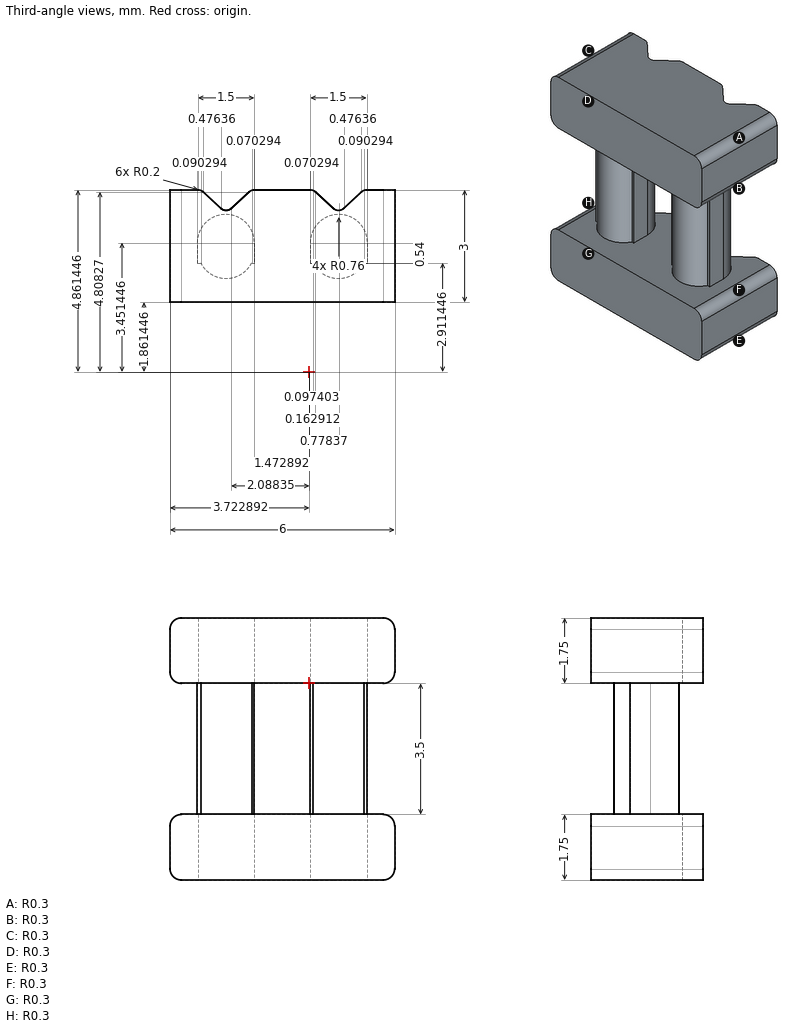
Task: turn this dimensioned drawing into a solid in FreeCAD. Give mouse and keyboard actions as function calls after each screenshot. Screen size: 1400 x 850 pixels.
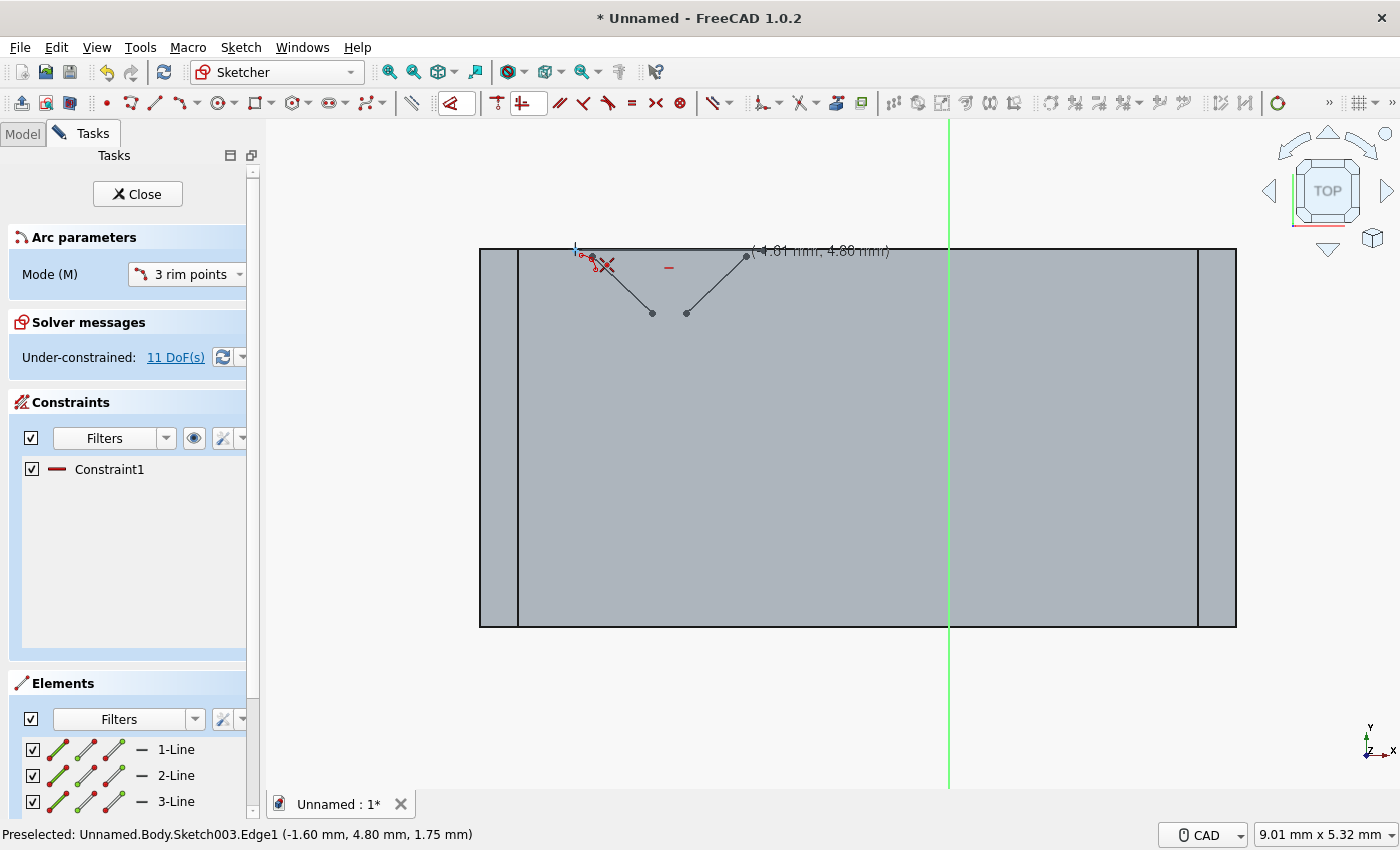
click(576, 250)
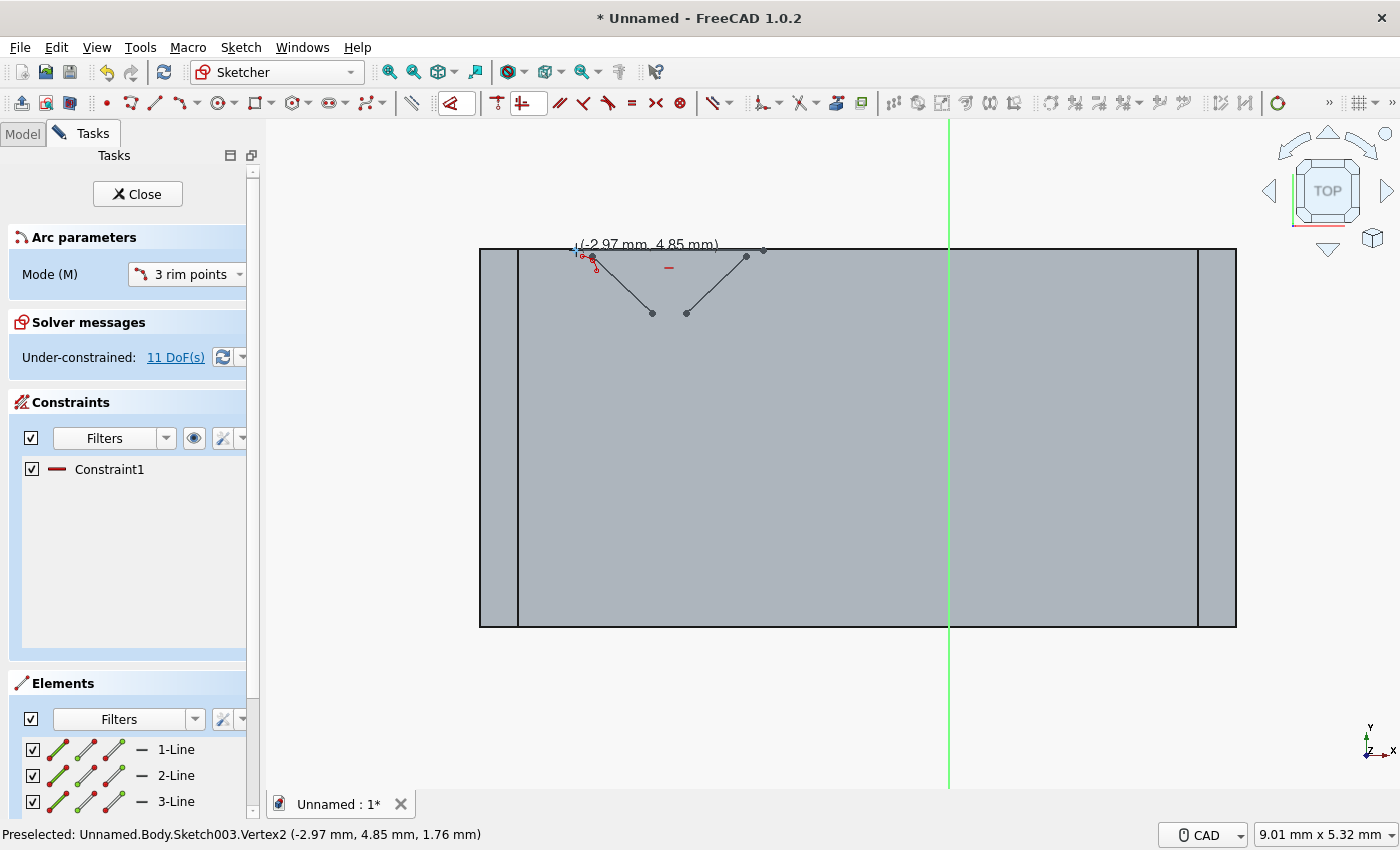
scroll(592, 256, up, 5)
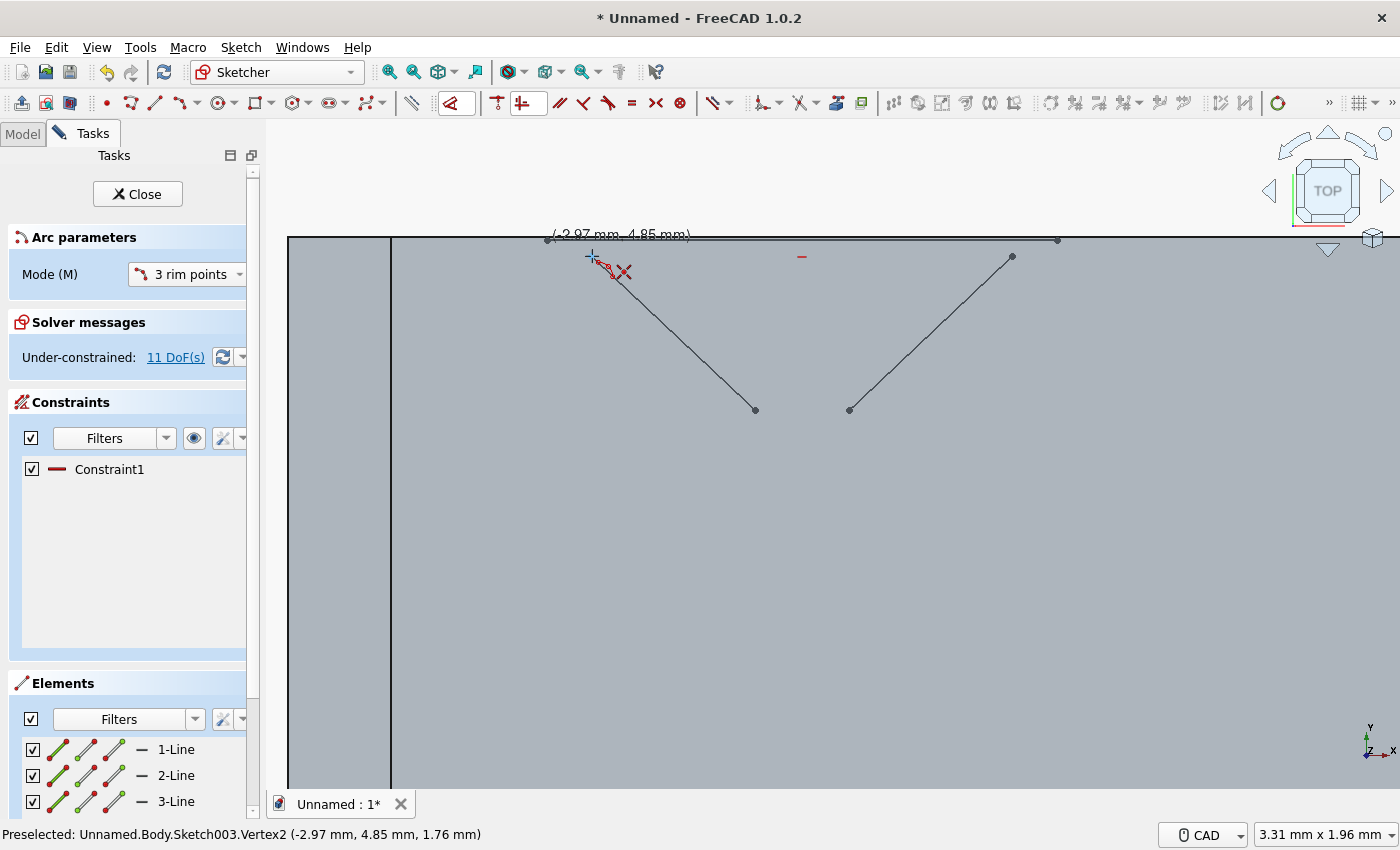
click(592, 256)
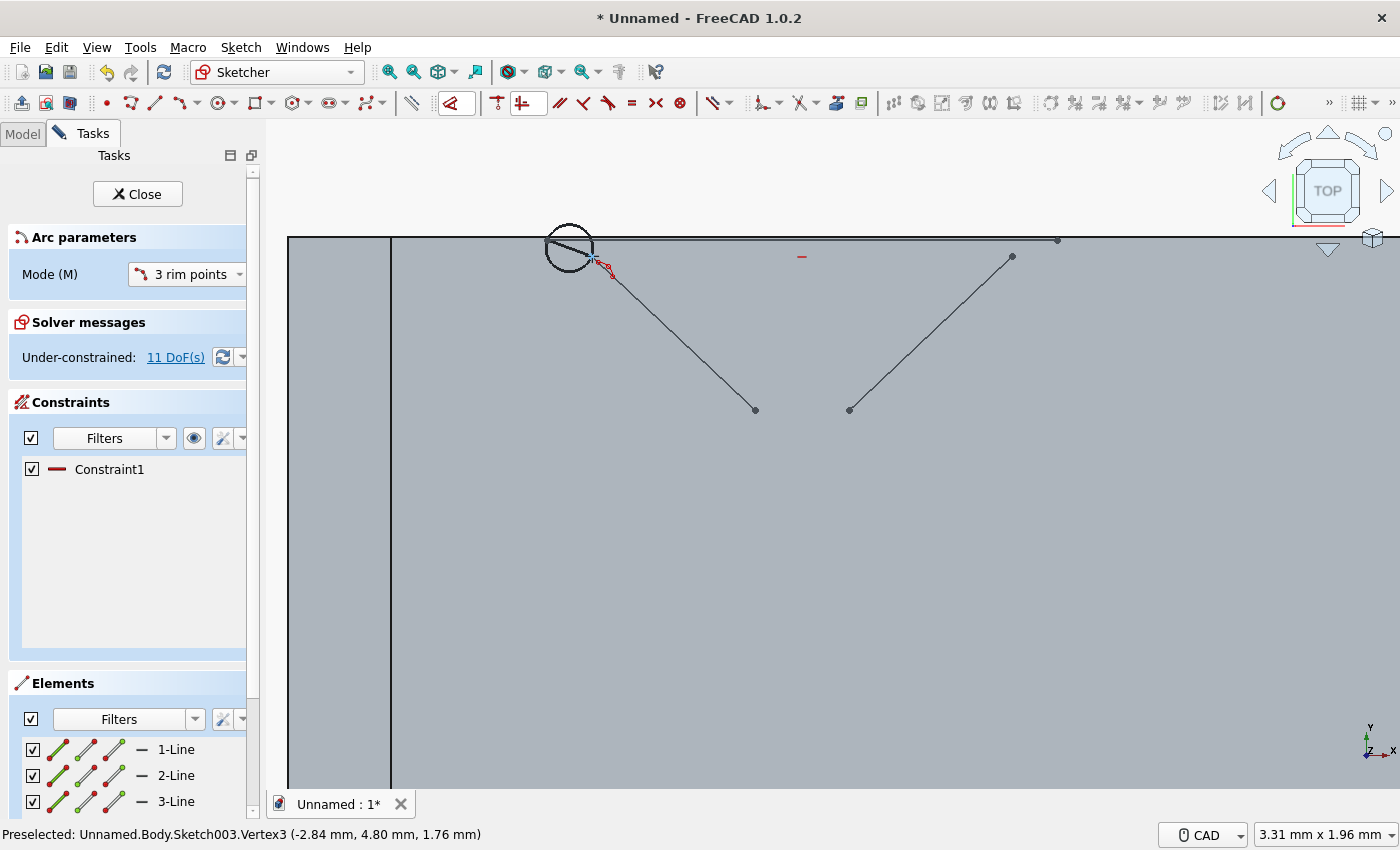
scroll(570, 242, up, 7)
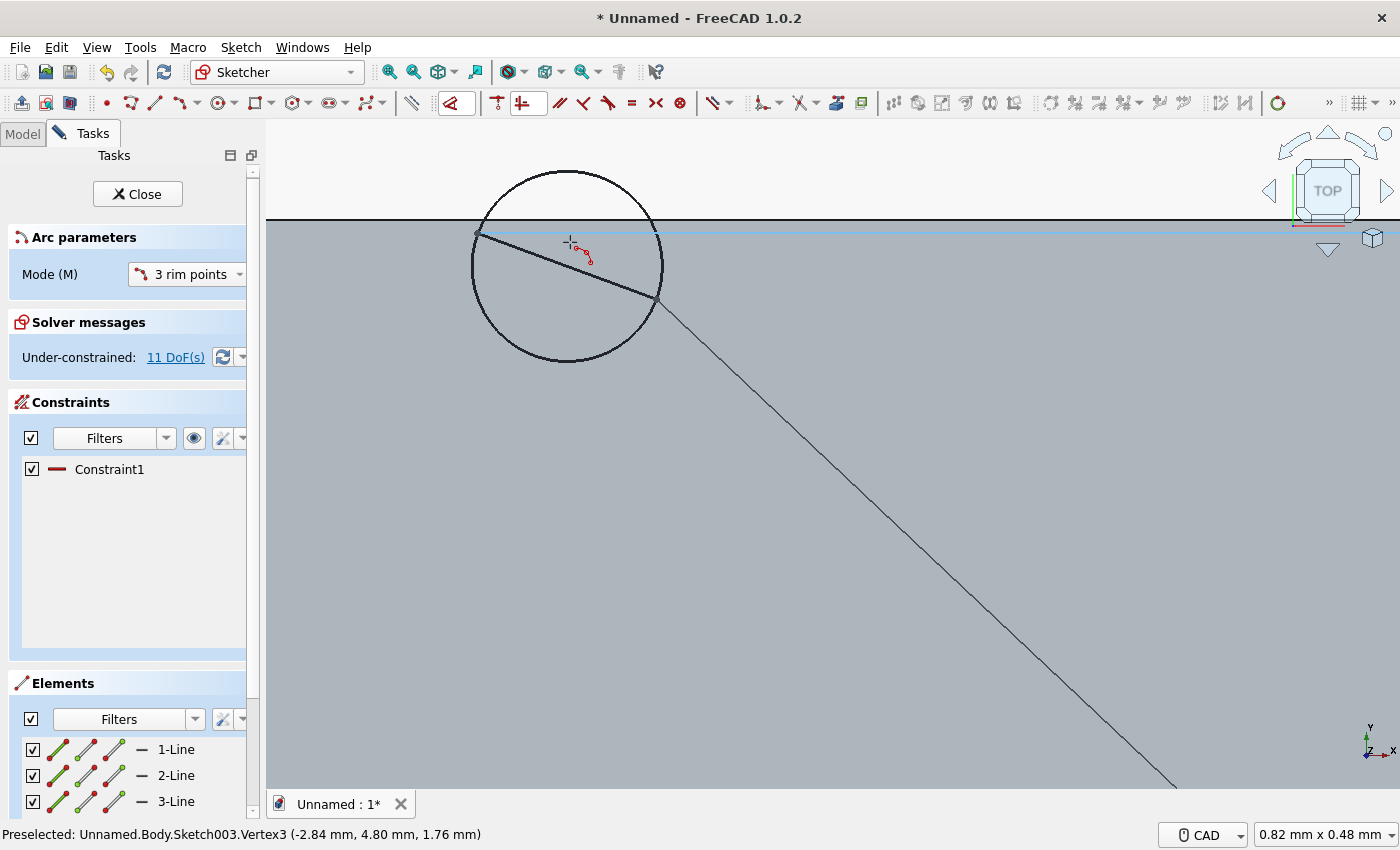
click(570, 239)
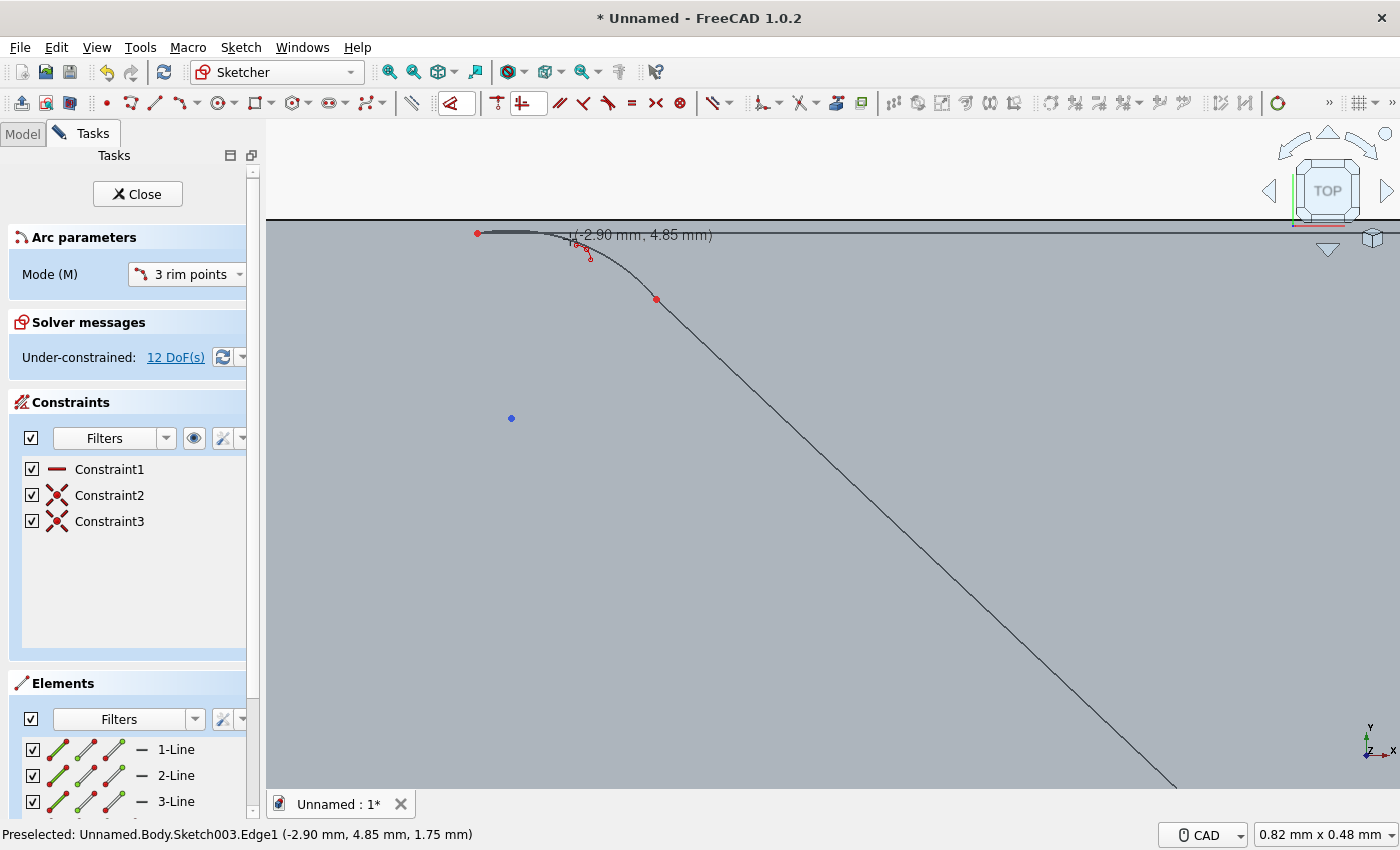
scroll(581, 251, down, 14)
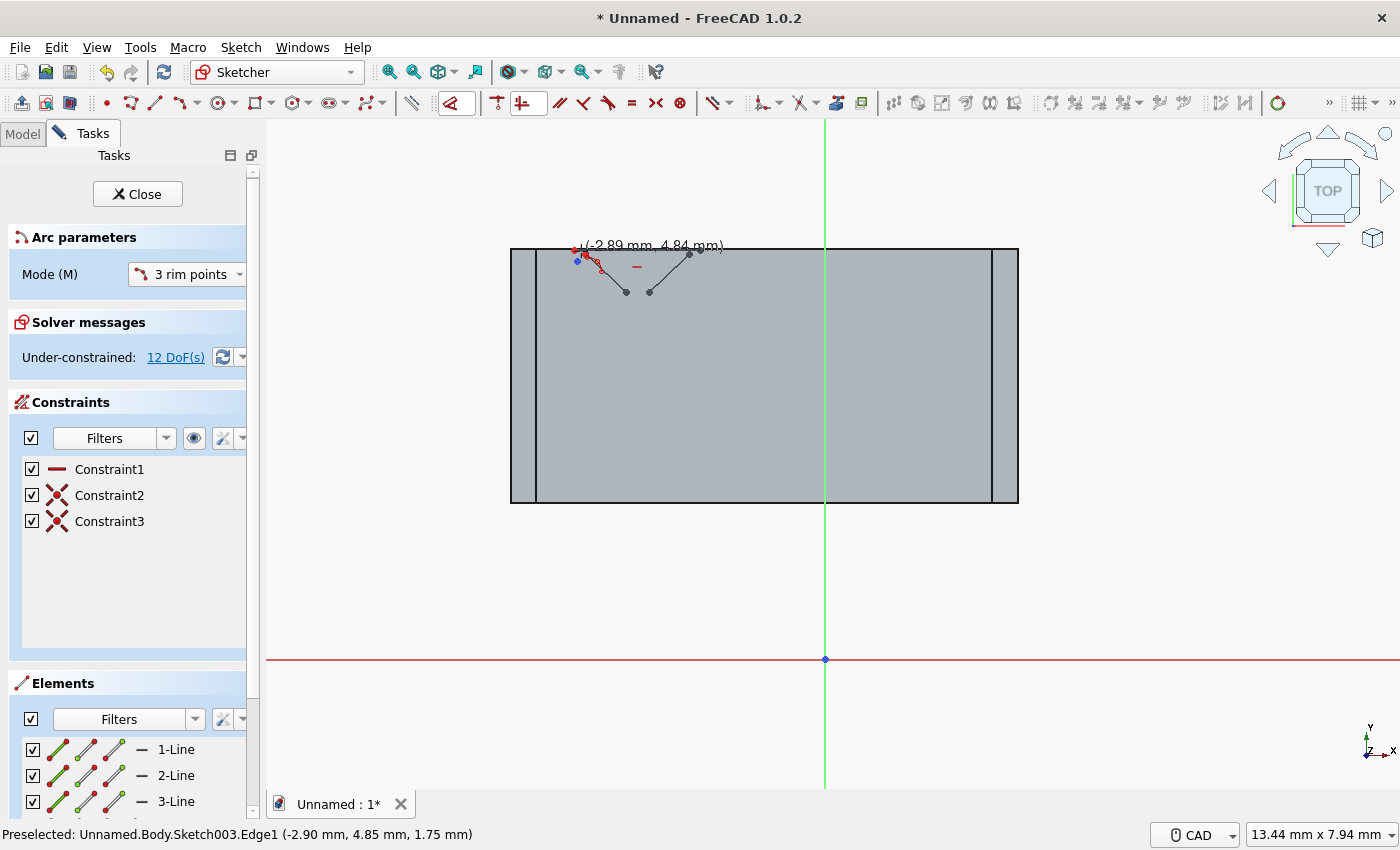
click(626, 292)
click(649, 292)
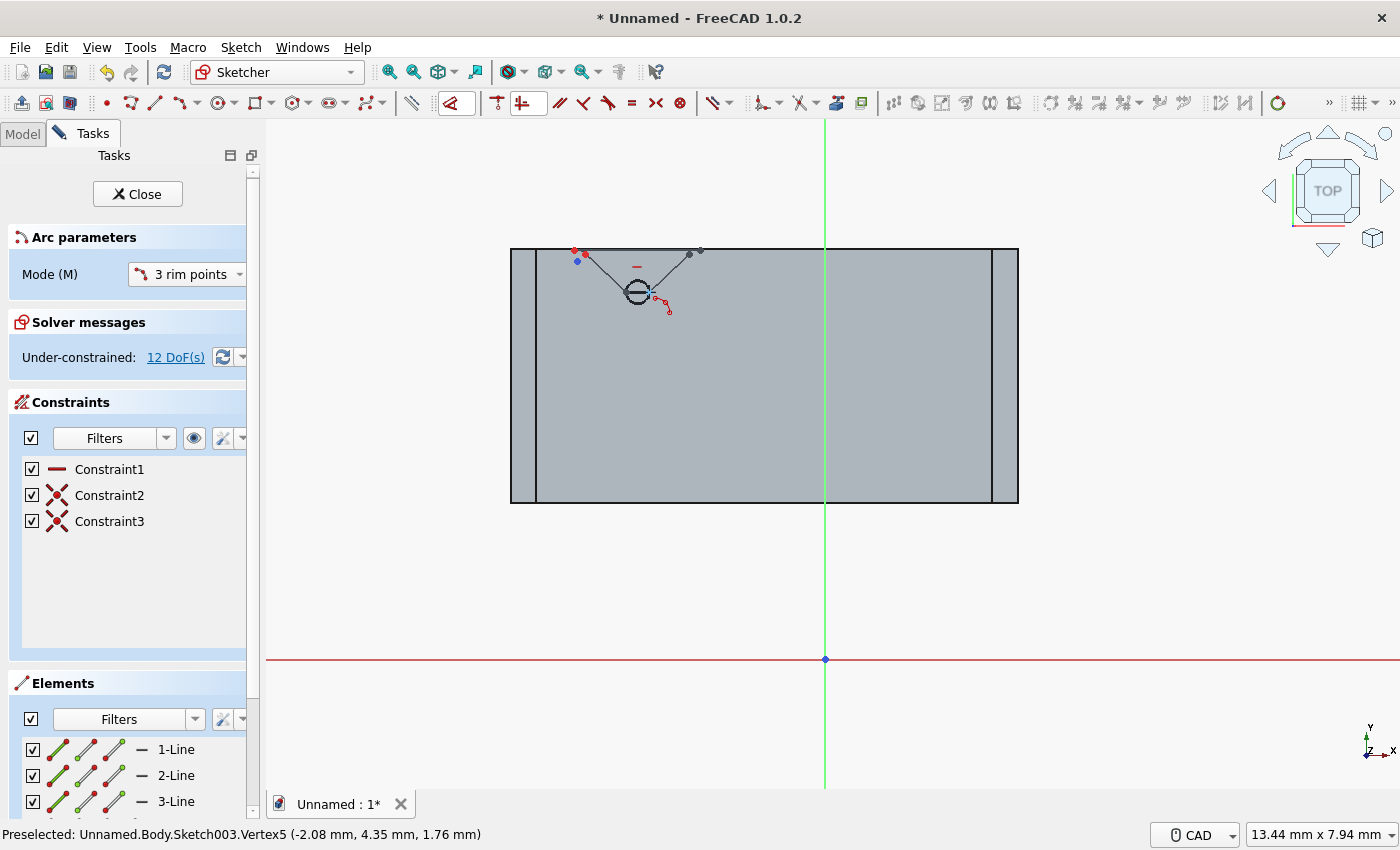
scroll(638, 296, up, 7)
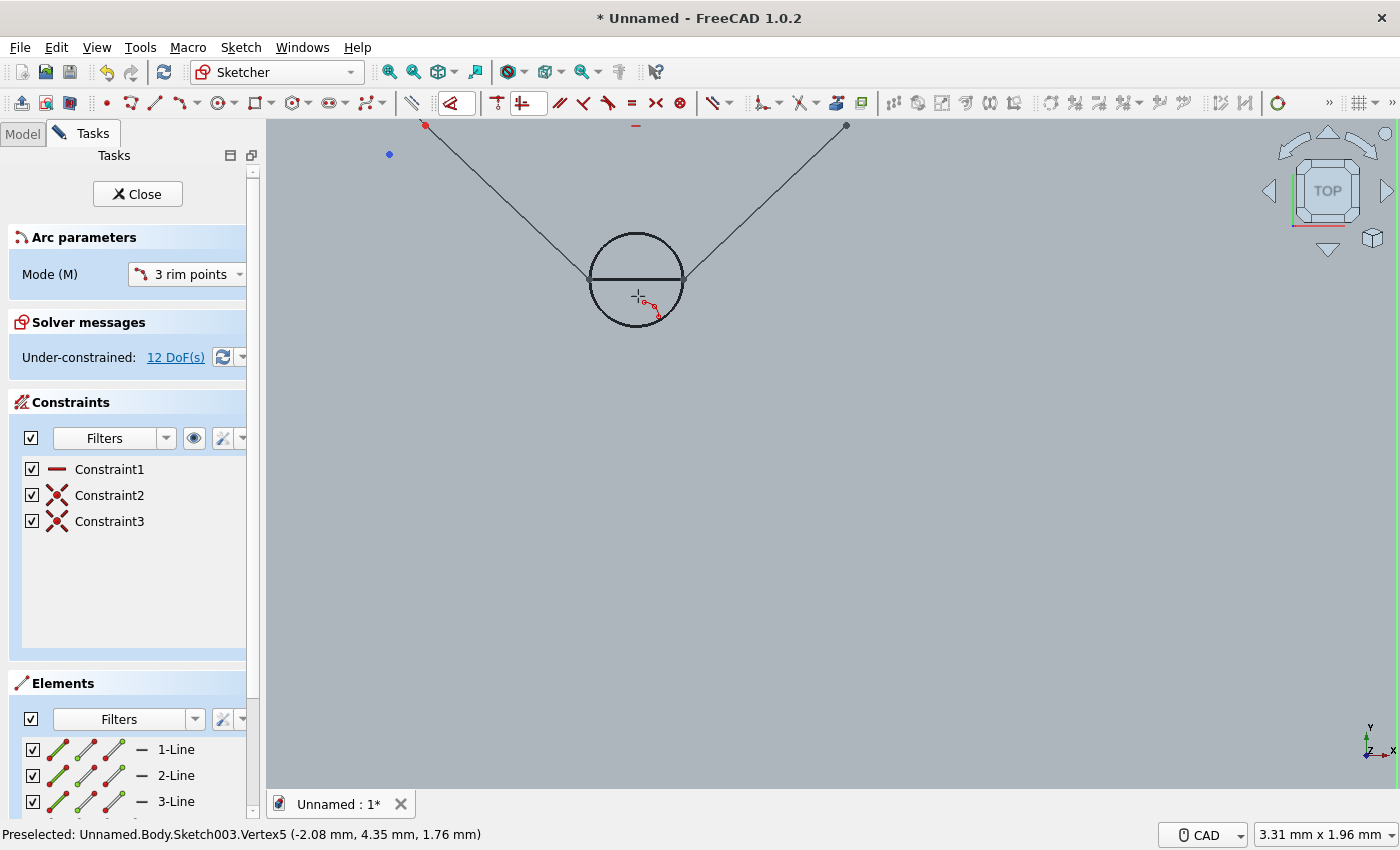
click(635, 294)